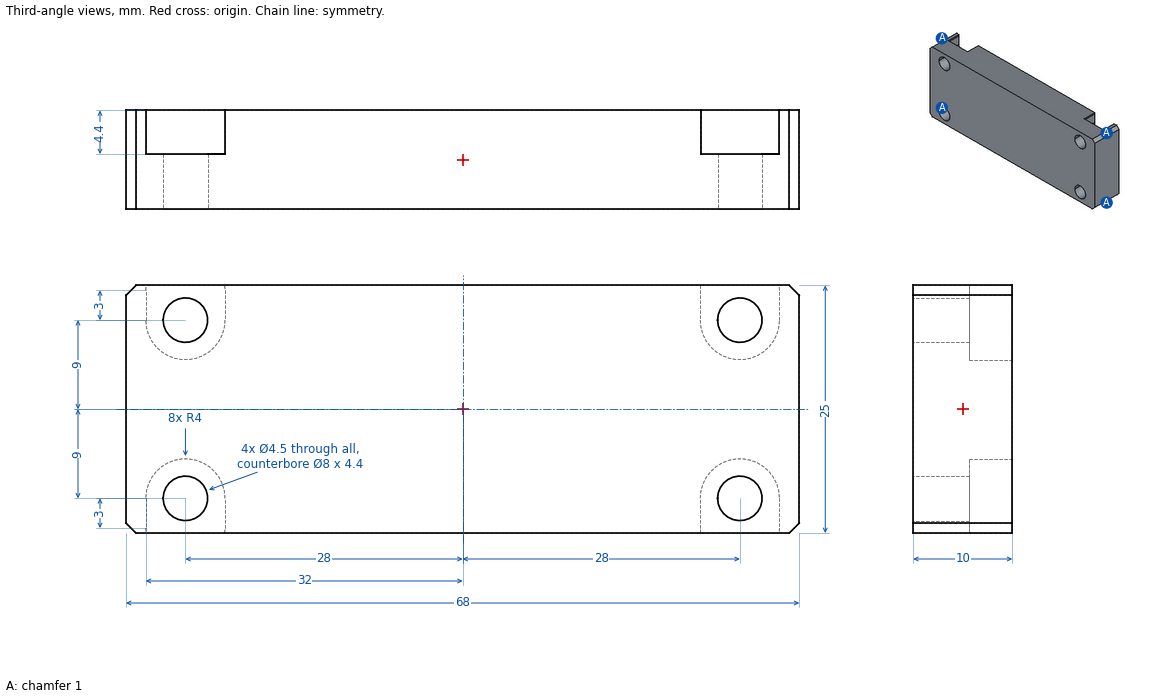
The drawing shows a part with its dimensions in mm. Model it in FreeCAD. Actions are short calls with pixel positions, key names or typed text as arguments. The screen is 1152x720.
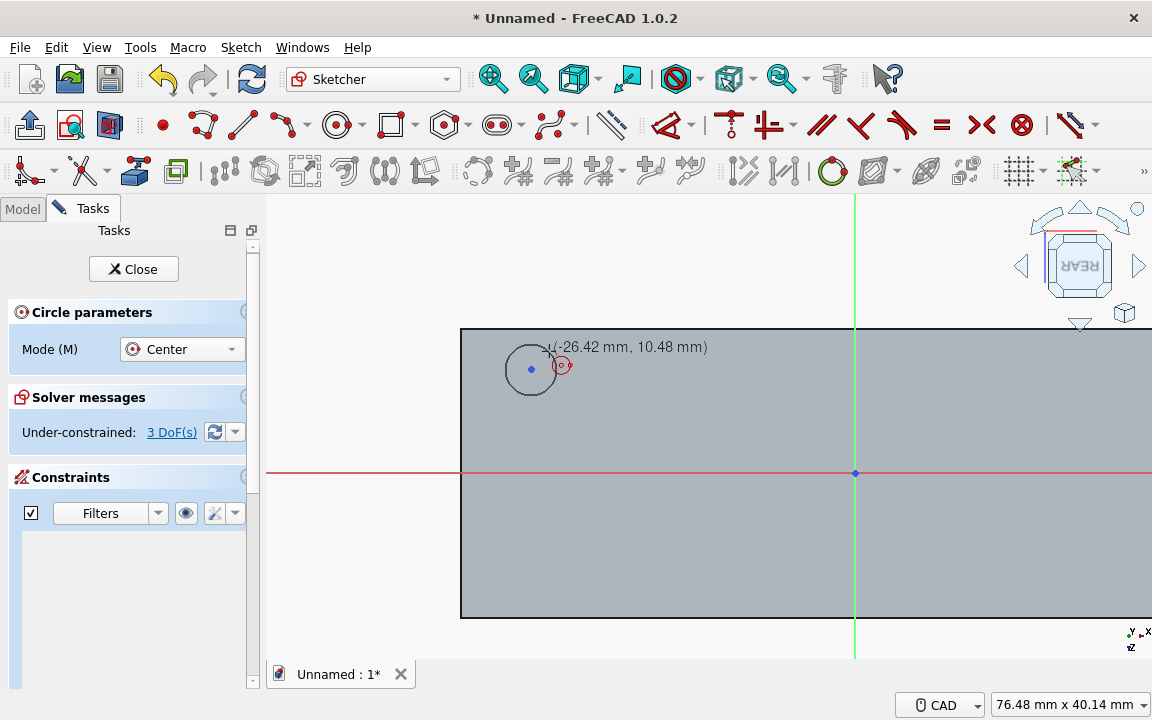
click(531, 578)
click(549, 559)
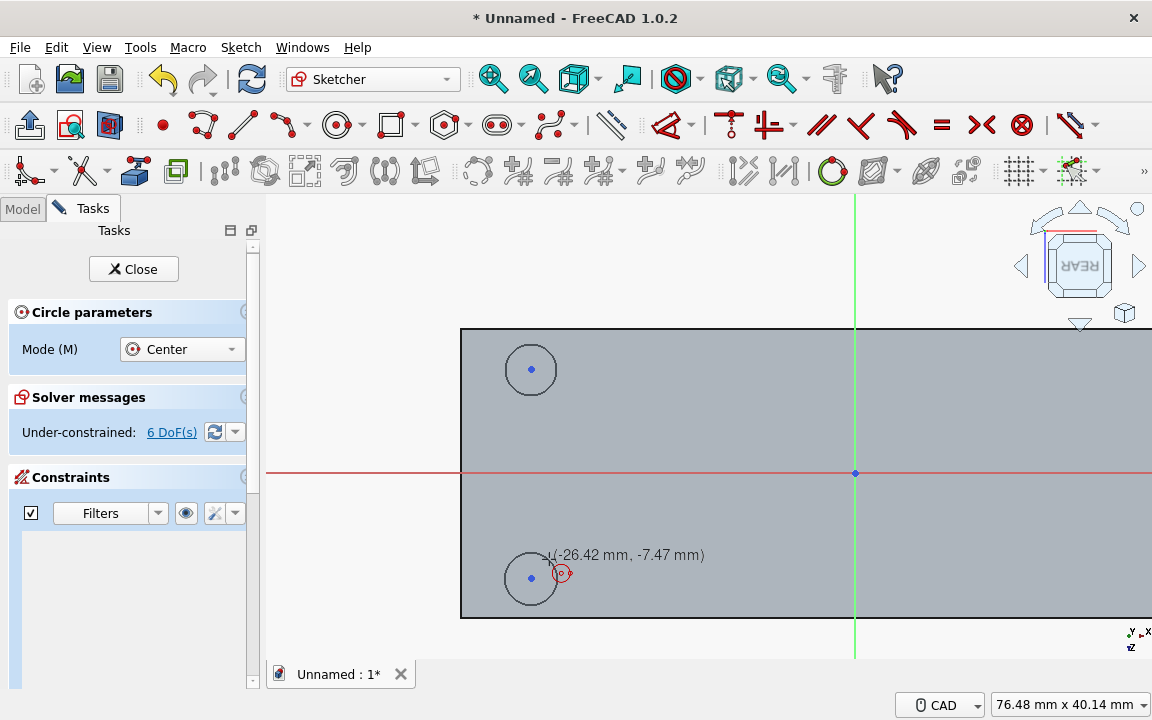
scroll(294, 331, down, 2)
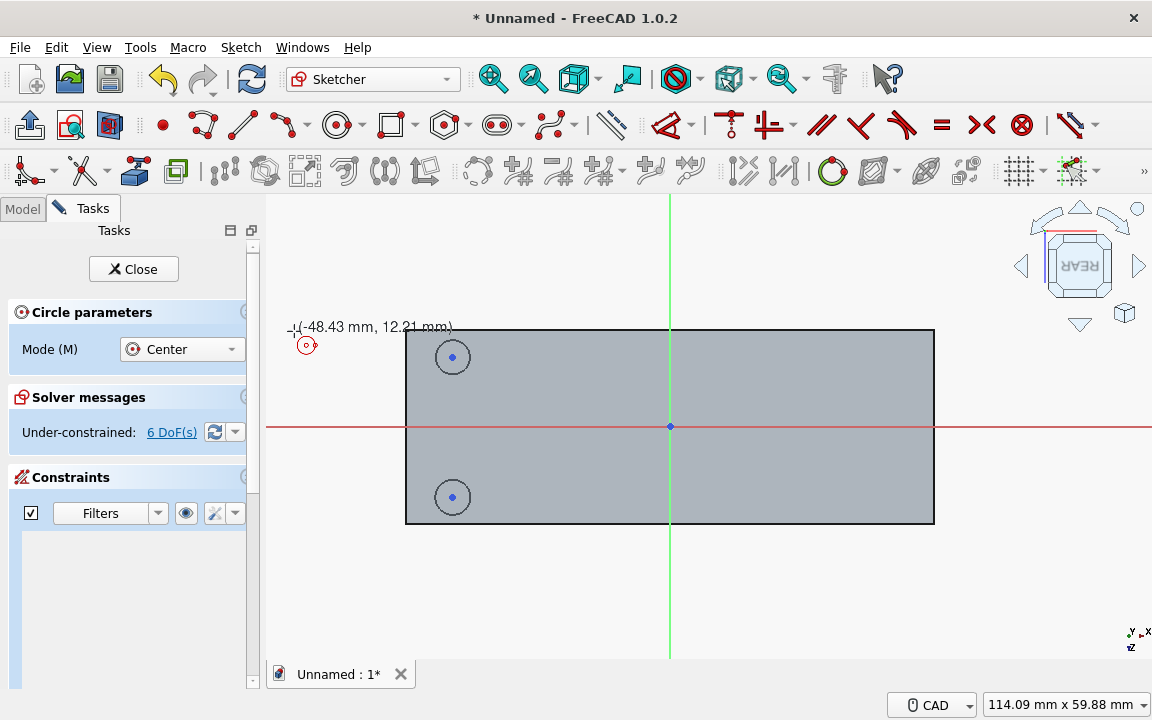
scroll(888, 357, up, 2)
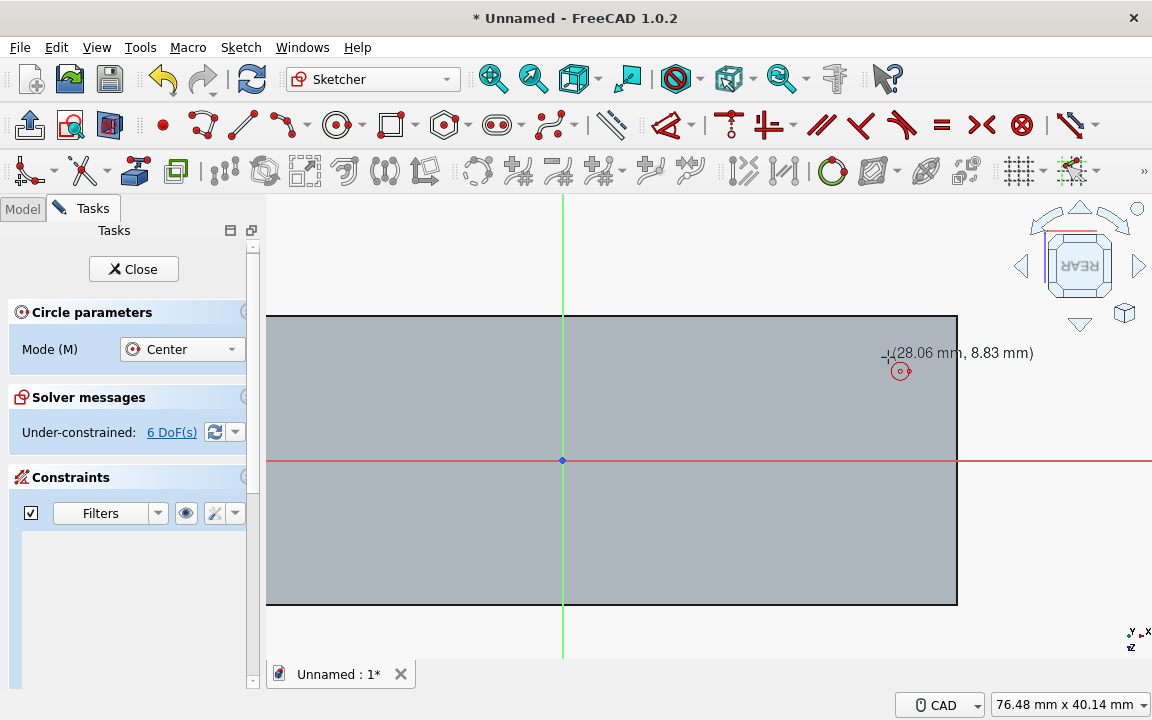
click(887, 356)
click(905, 338)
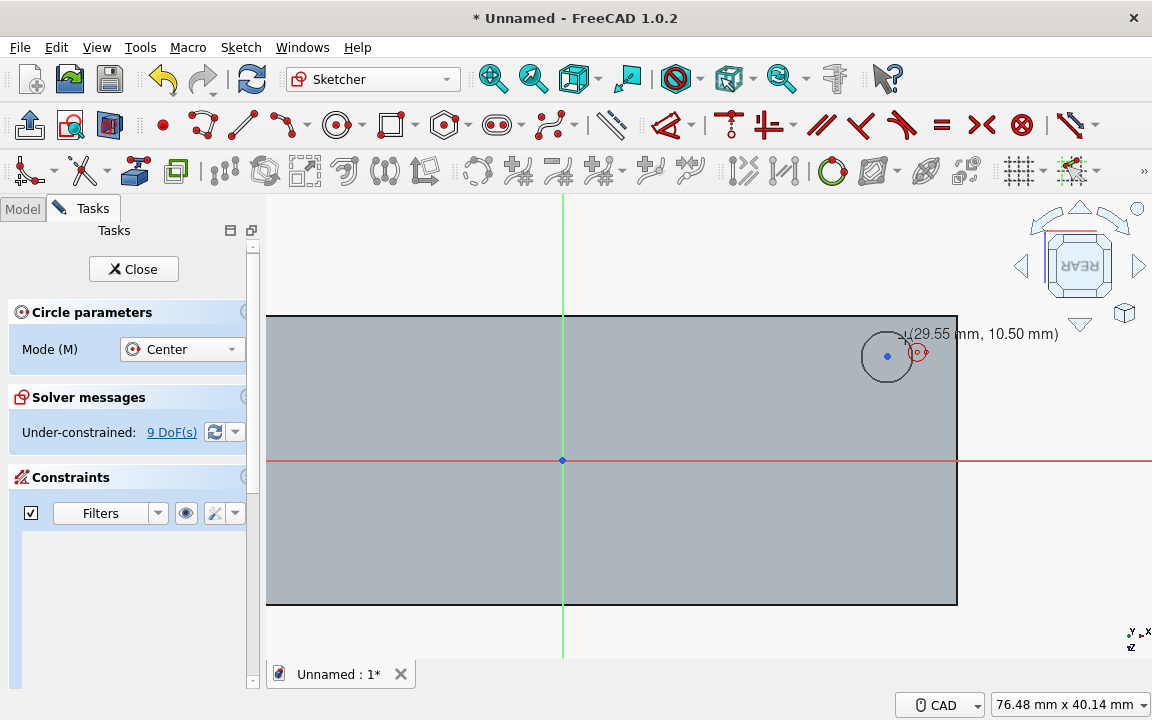
click(887, 565)
click(905, 546)
key(Escape)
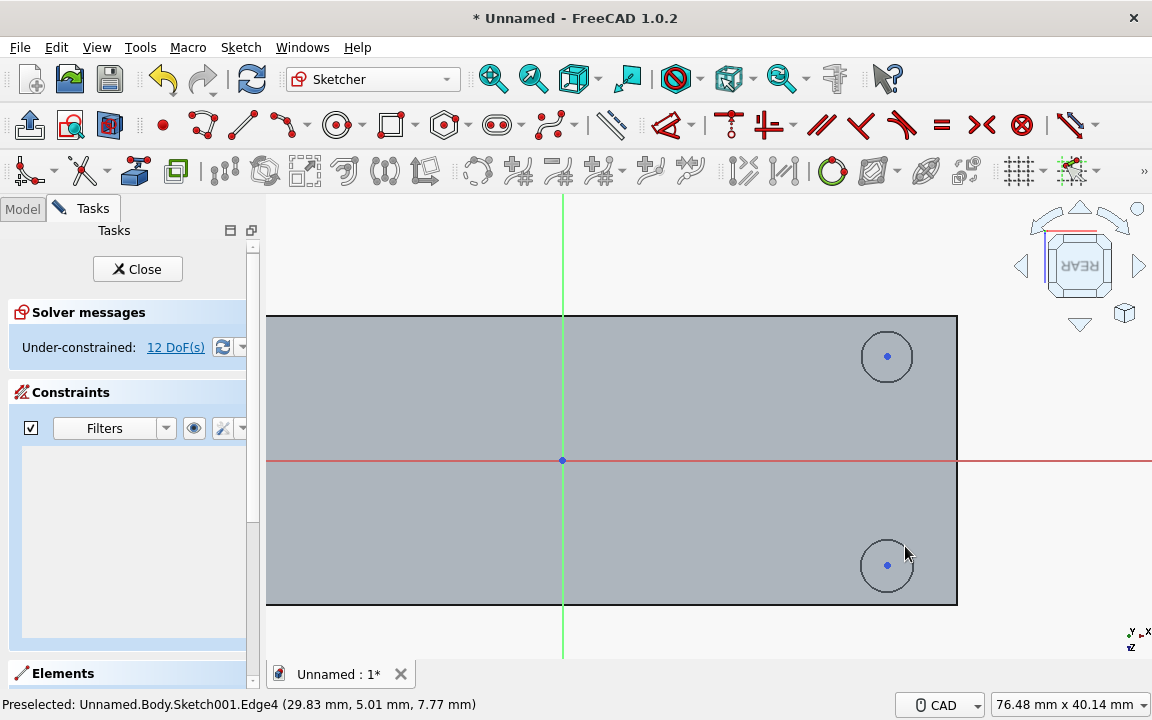
scroll(799, 357, down, 2)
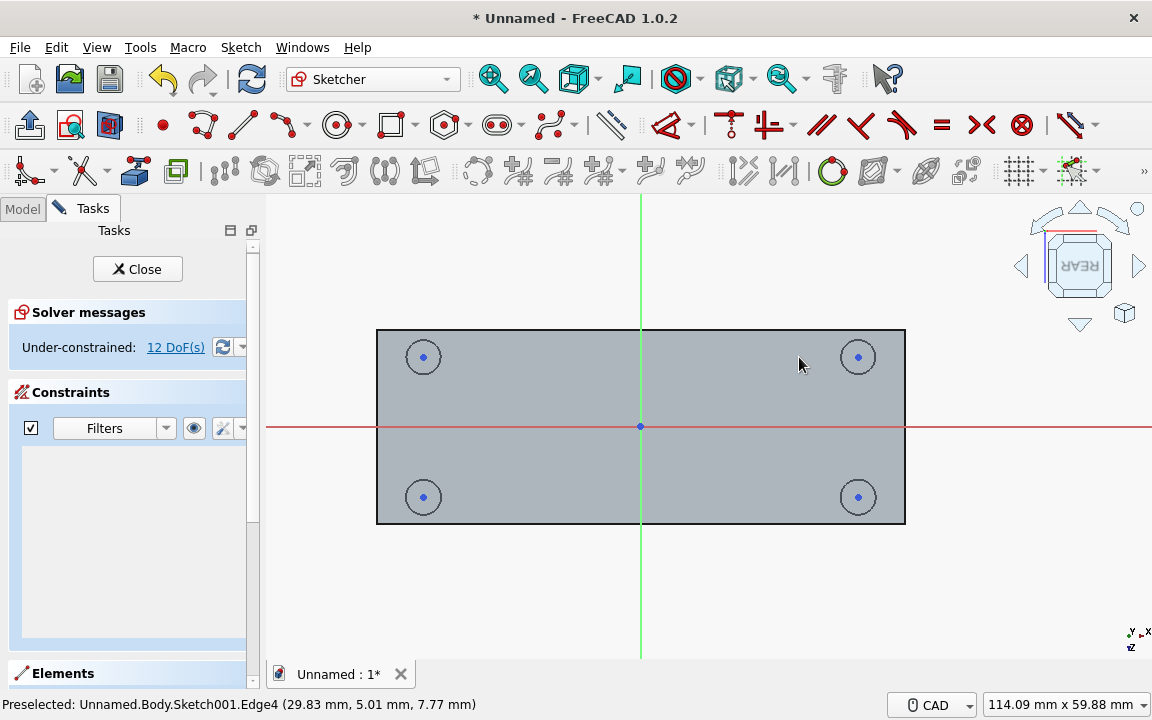
click(436, 345)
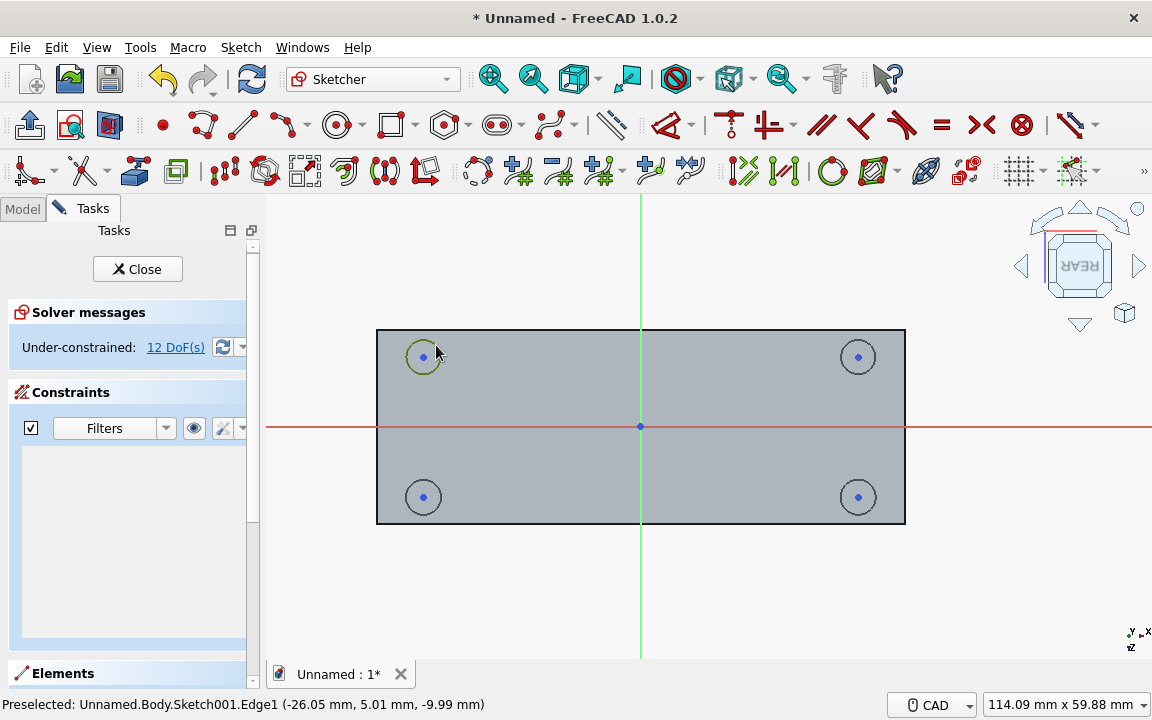
click(436, 485)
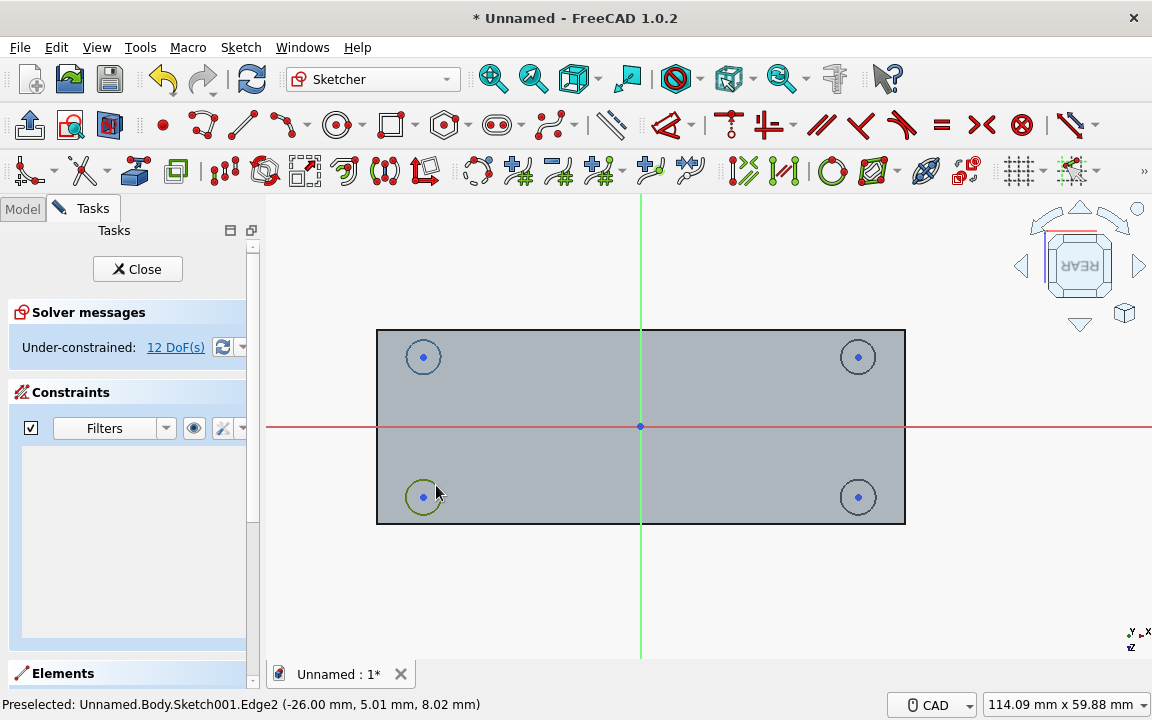
click(870, 345)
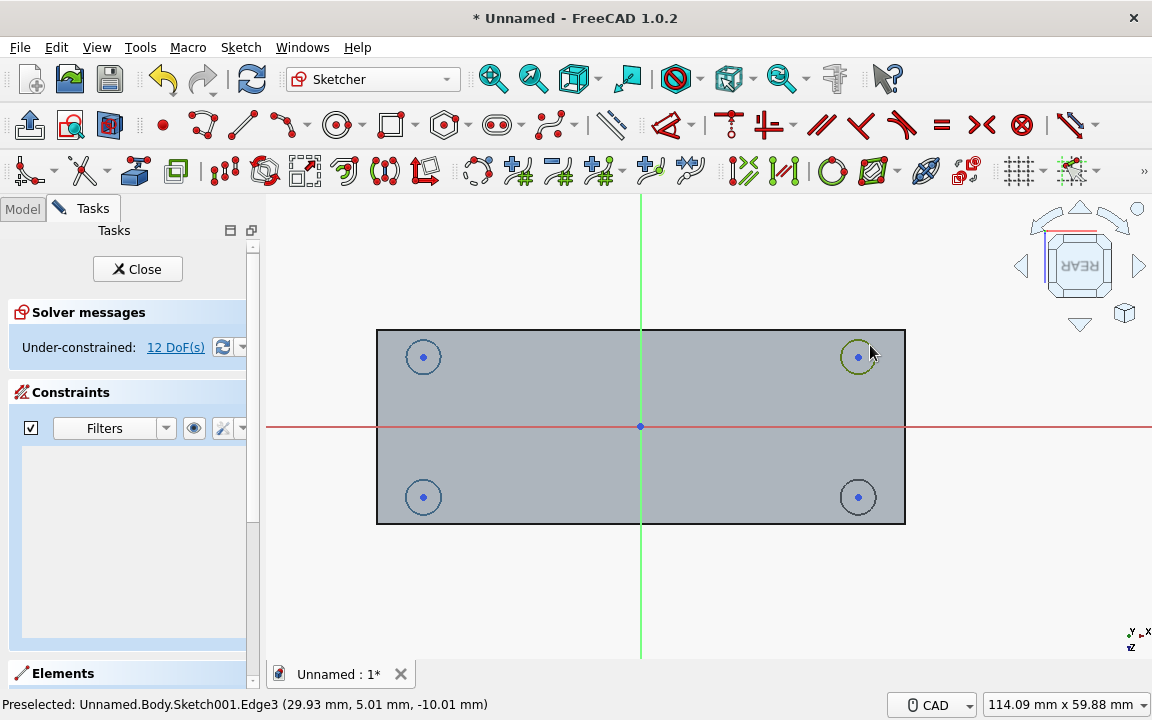
click(871, 485)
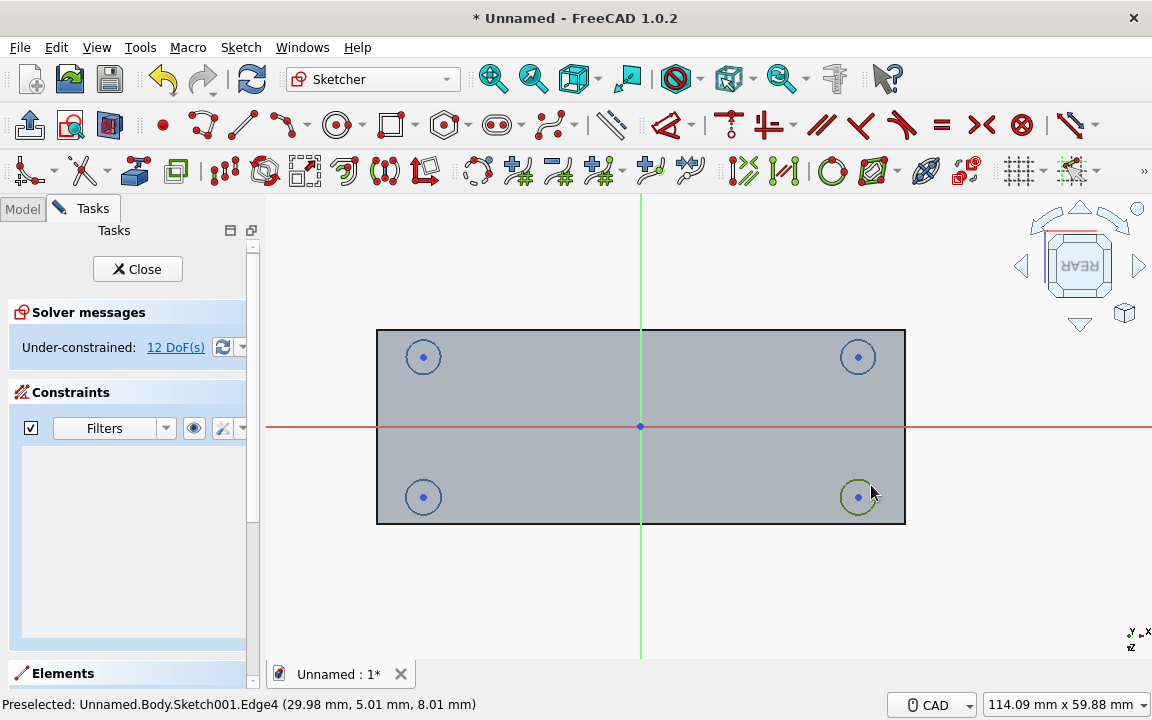
click(942, 126)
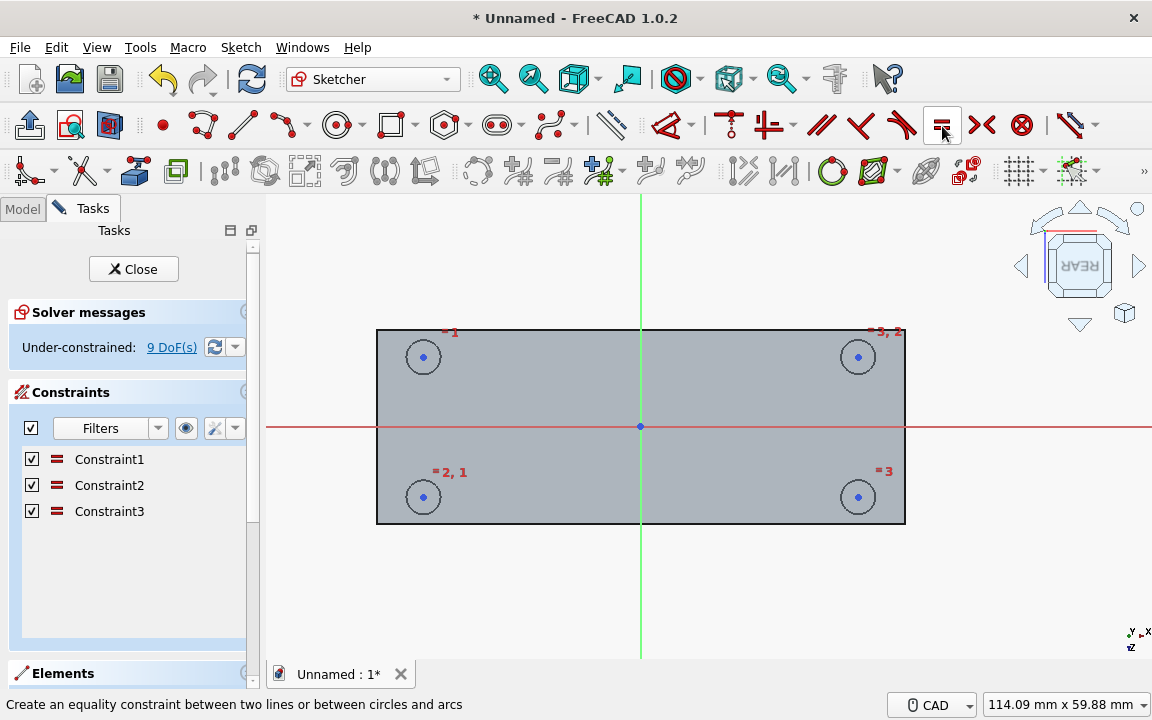
click(424, 357)